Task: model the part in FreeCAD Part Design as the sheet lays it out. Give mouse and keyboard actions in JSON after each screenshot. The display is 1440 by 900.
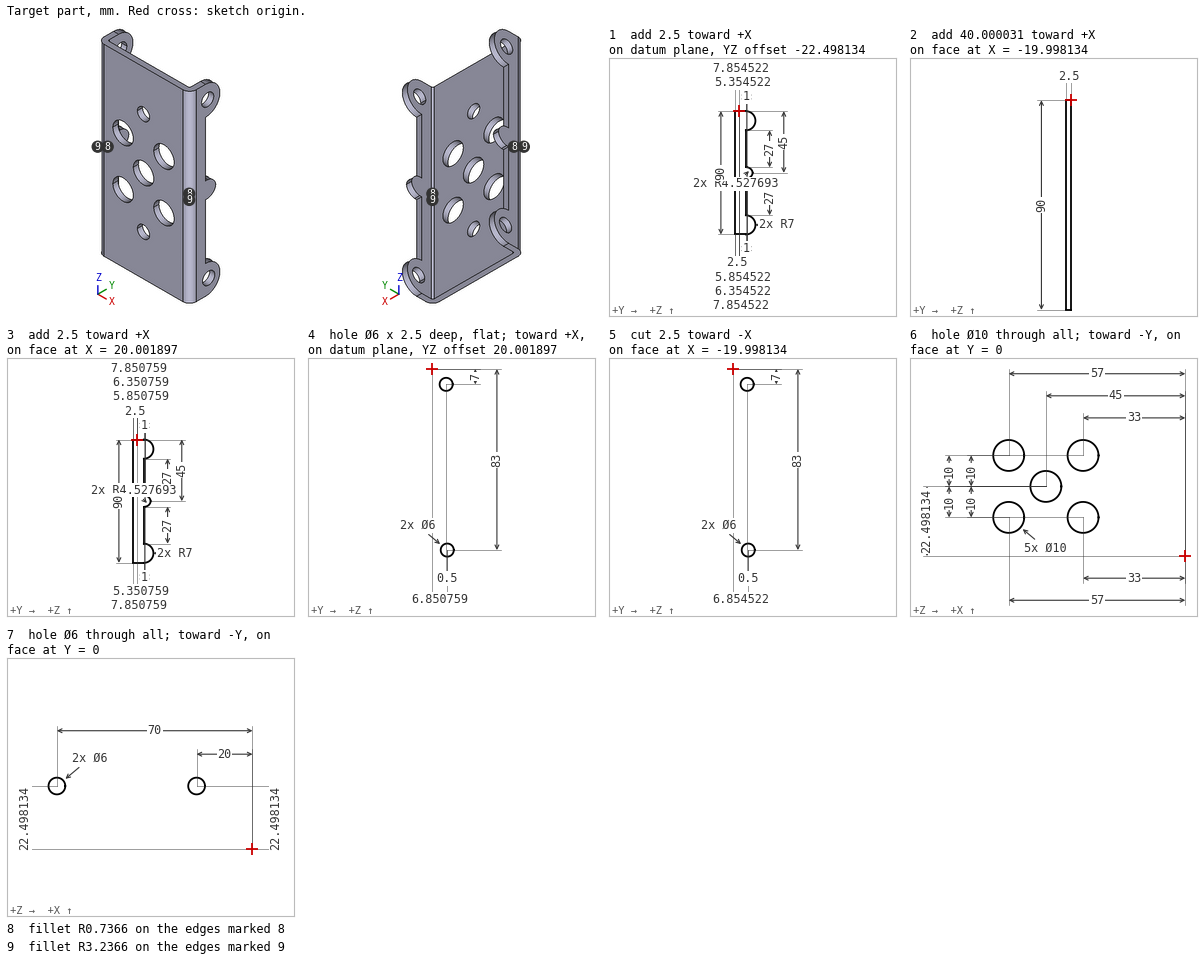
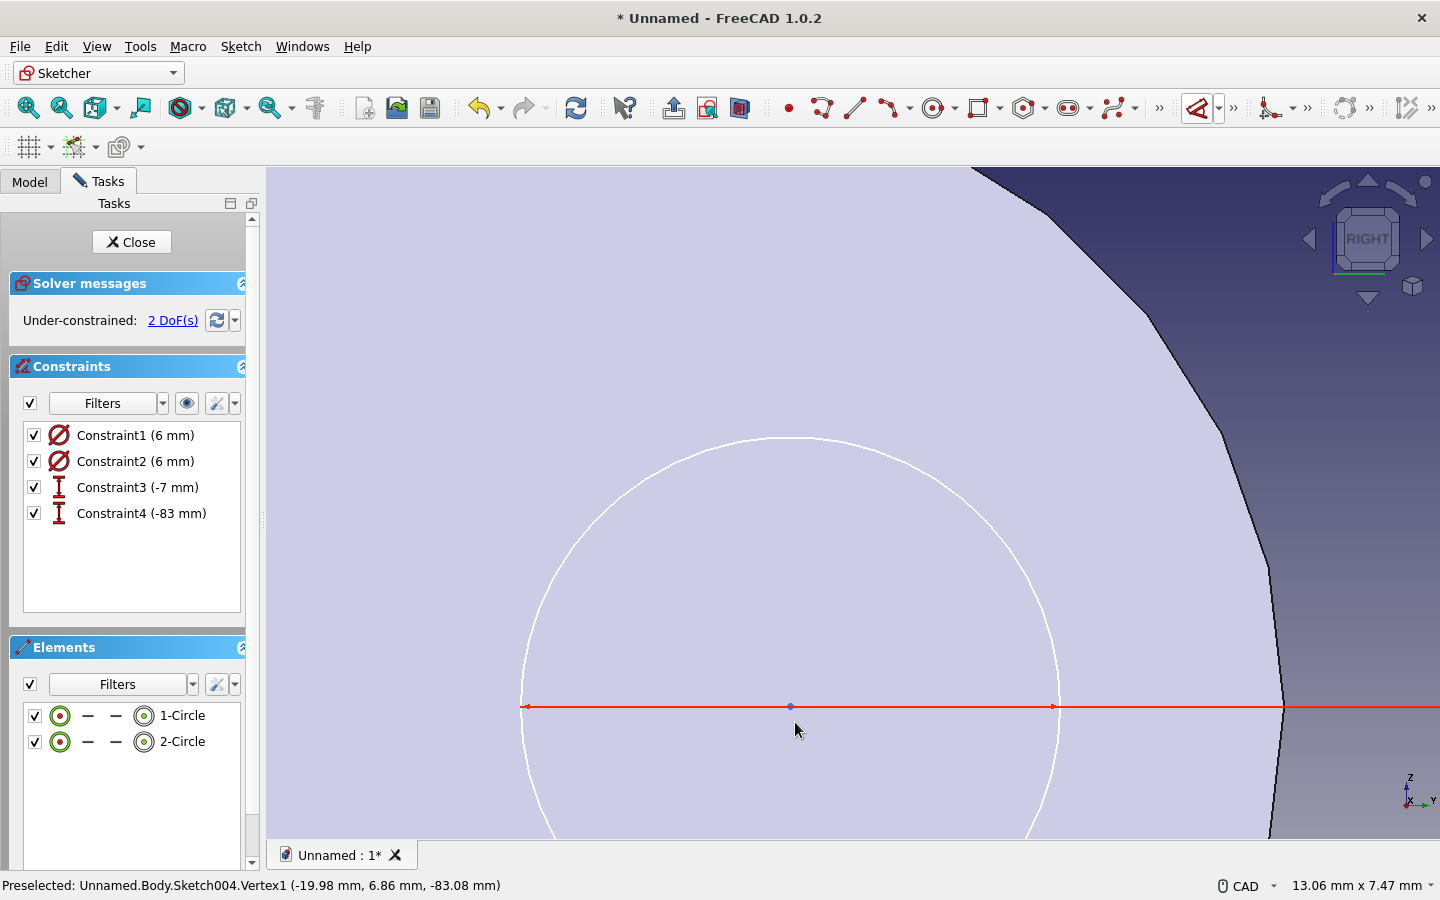
{"action": "left_click", "coordinate": [790, 707]}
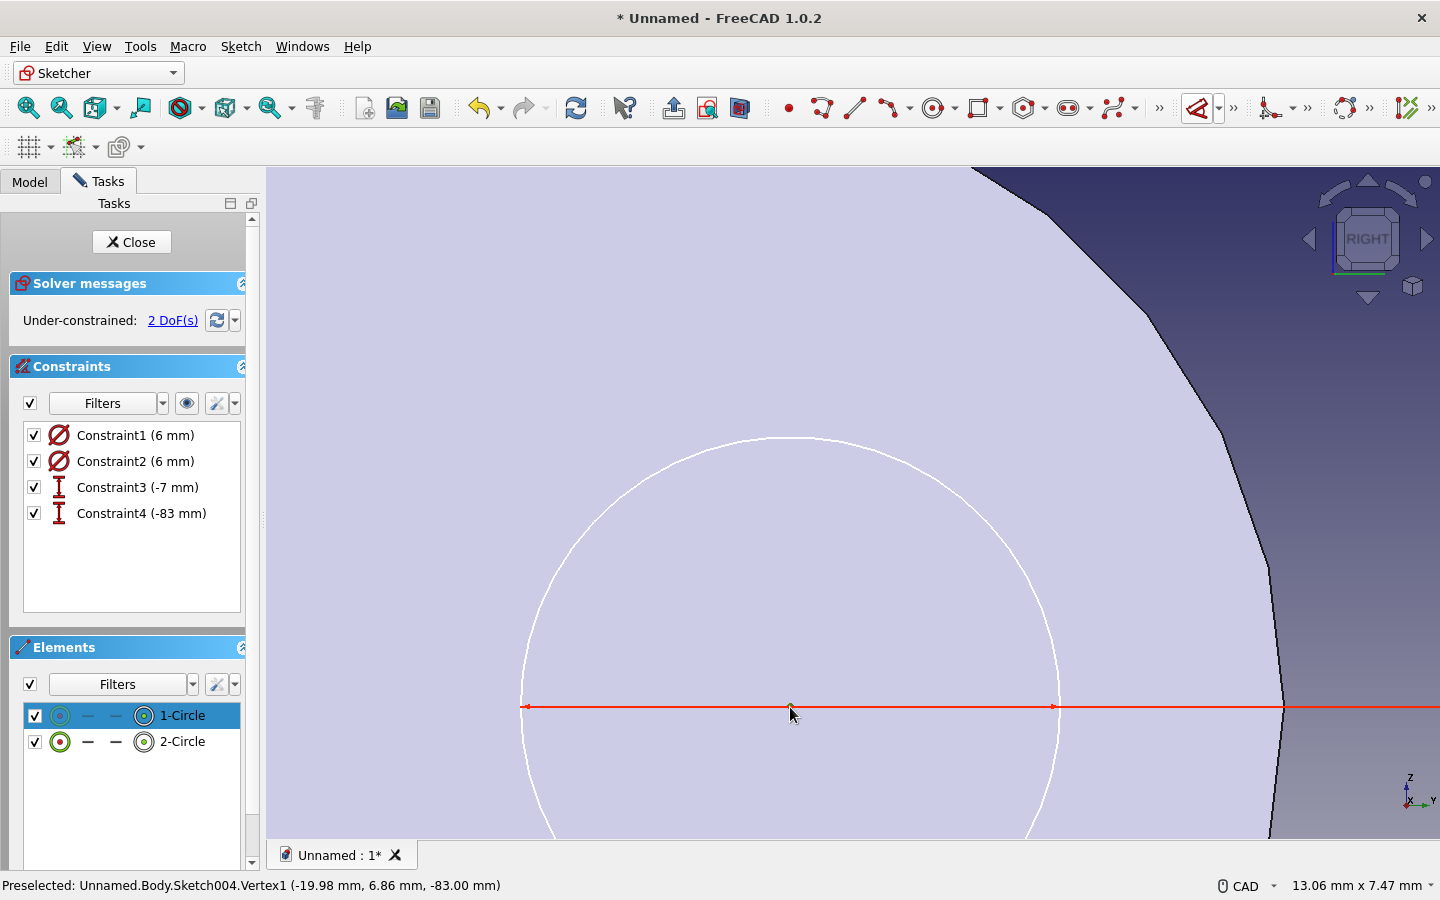
{"action": "scroll", "coordinate": [795, 723], "scroll_direction": "down", "scroll_amount": 14}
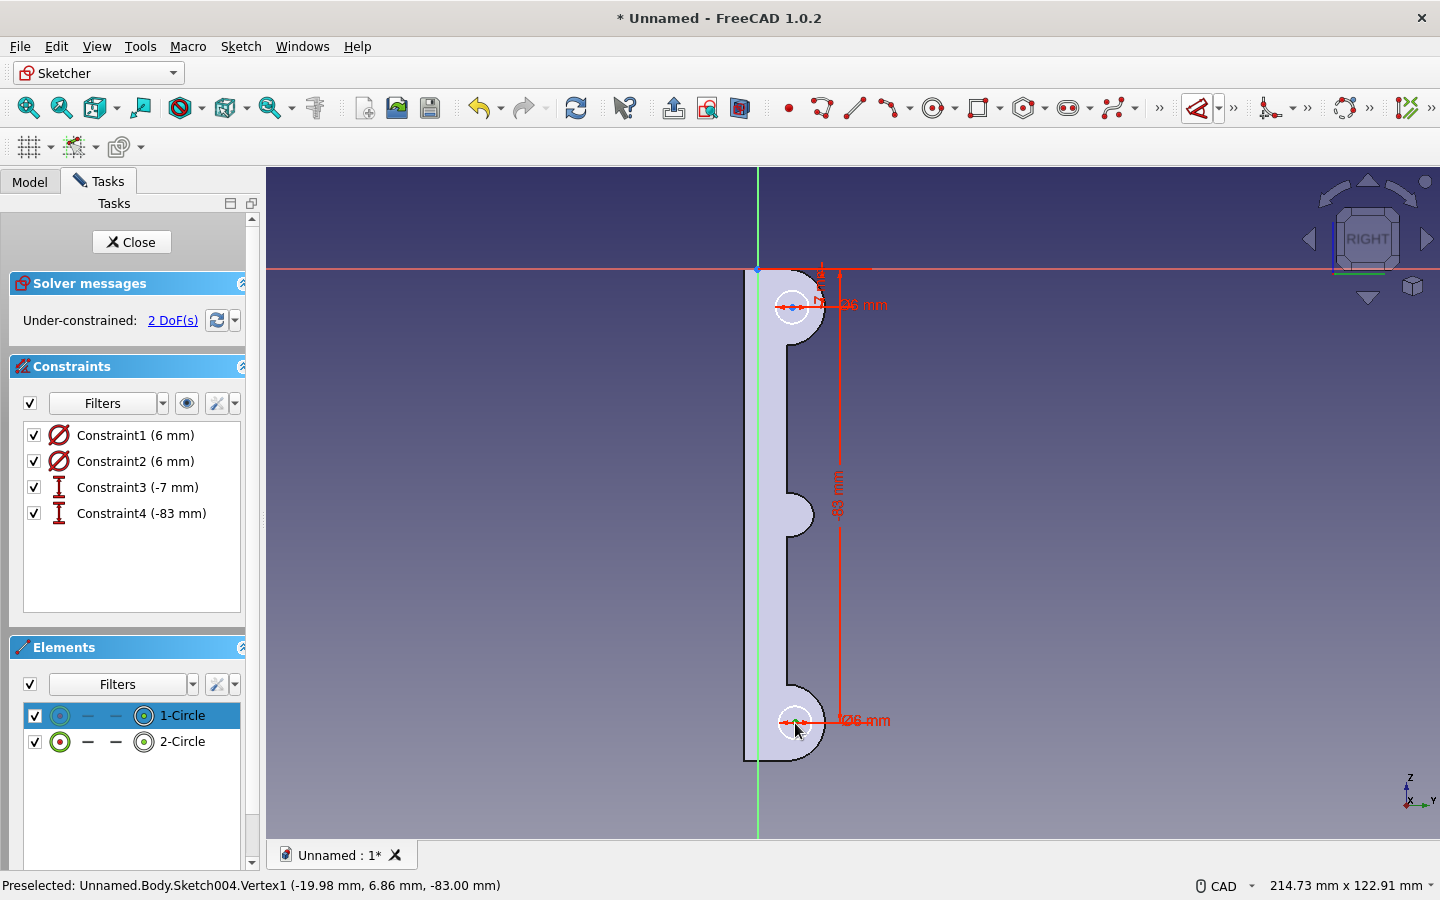
{"action": "scroll", "coordinate": [792, 307], "scroll_direction": "up", "scroll_amount": 14}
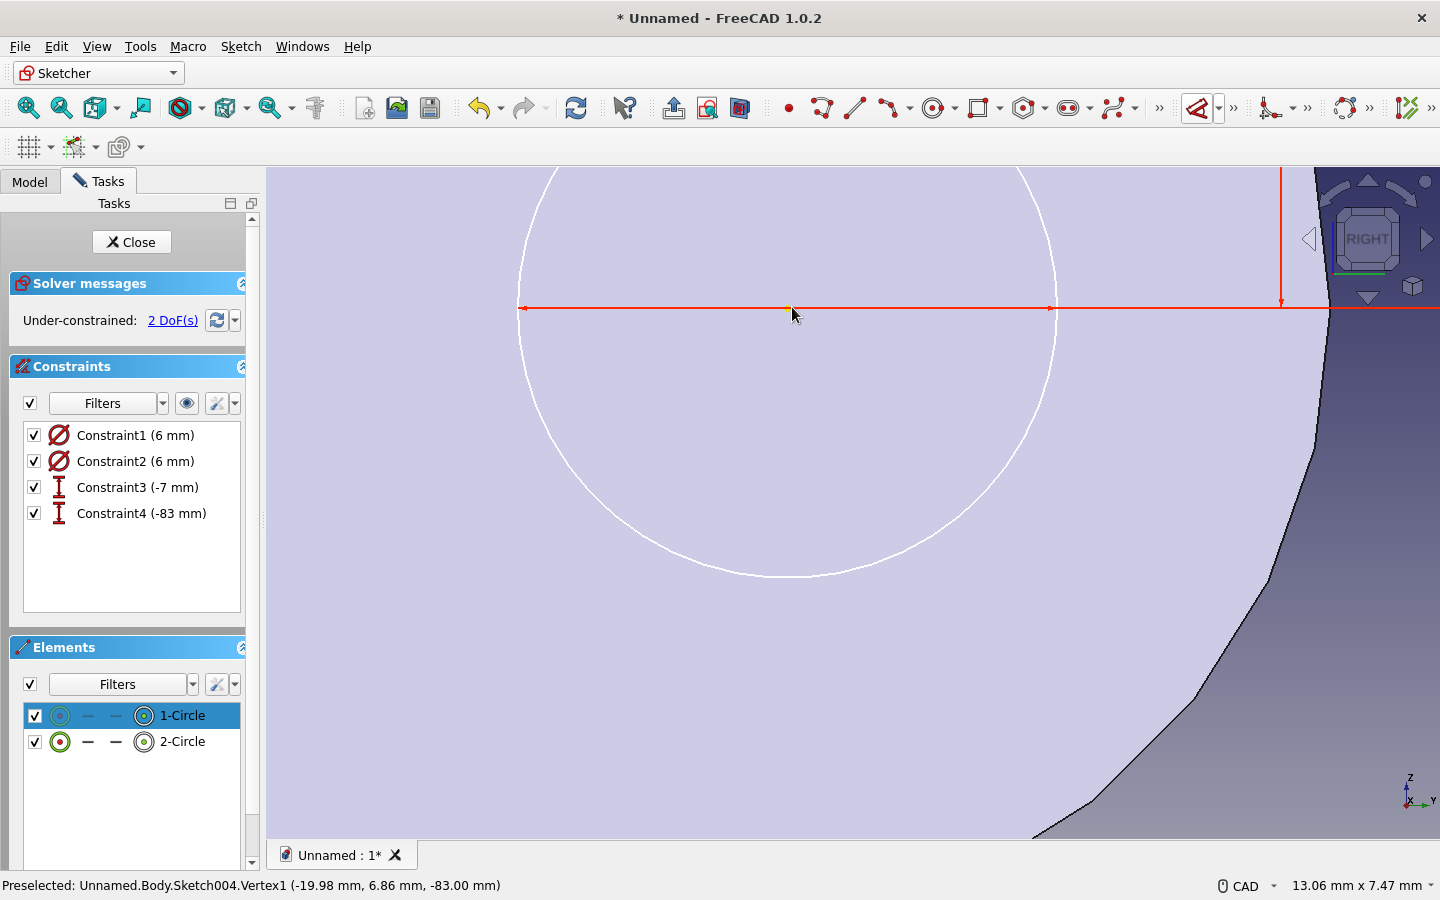
{"action": "left_click", "coordinate": [788, 308]}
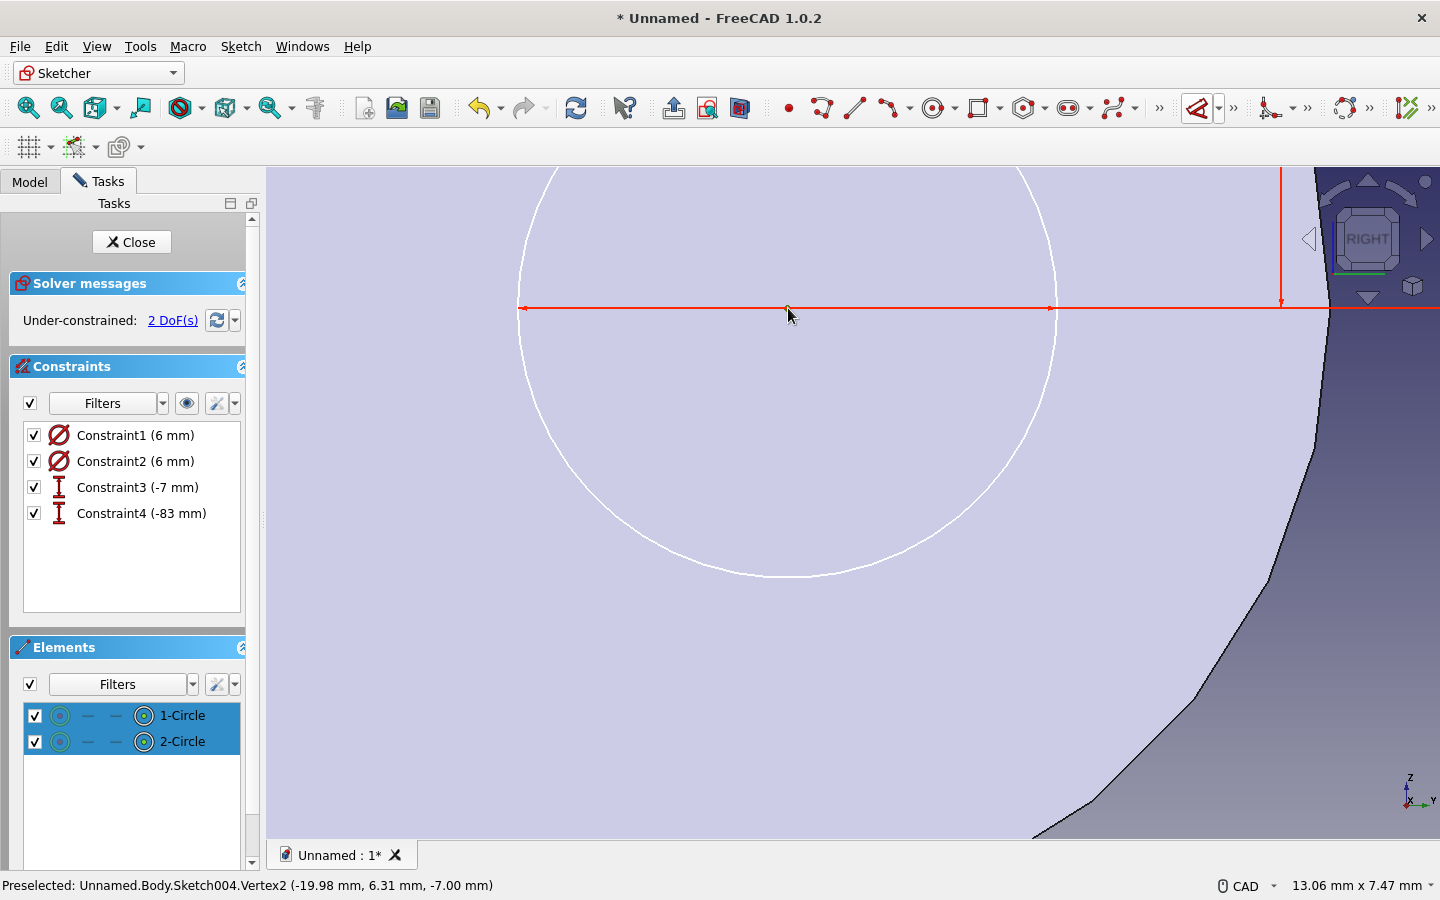
{"action": "left_click", "coordinate": [1218, 108]}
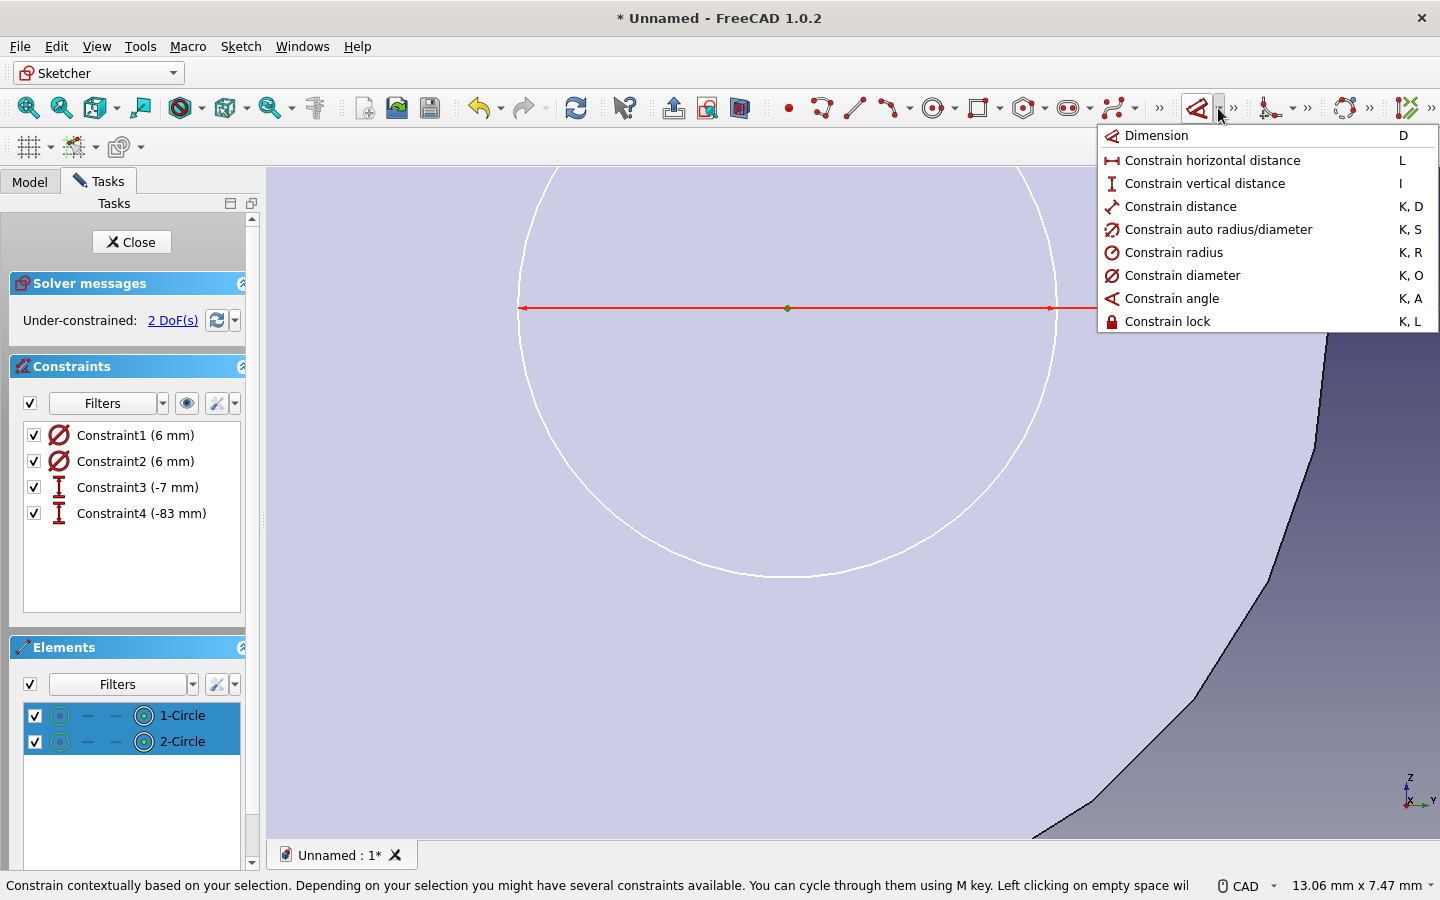
{"action": "left_click", "coordinate": [1268, 160]}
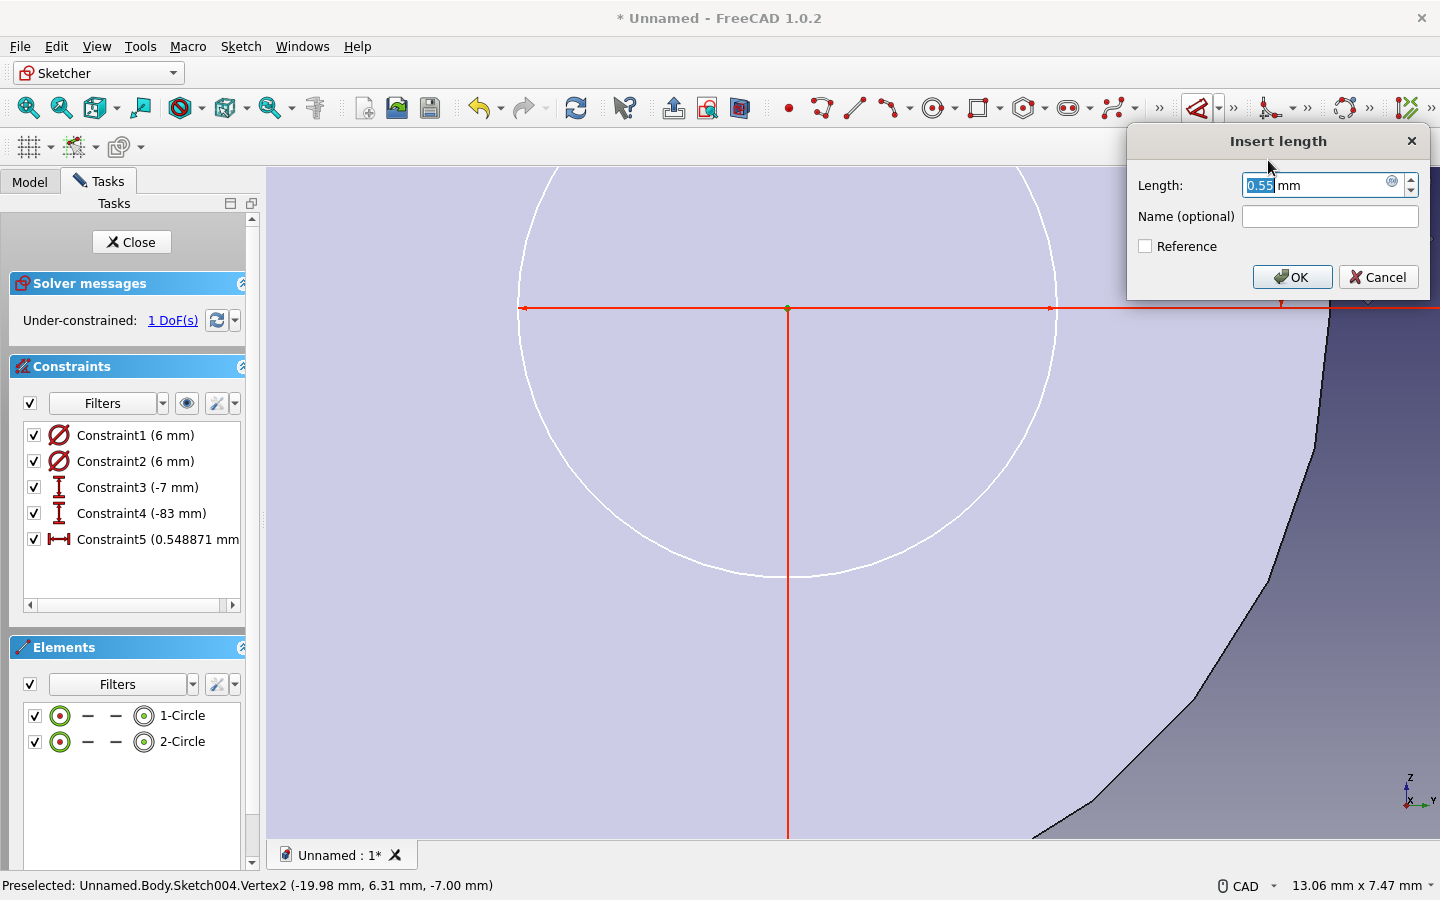
{"action": "type", "text": "0.5"}
{"action": "key", "text": "Return"}